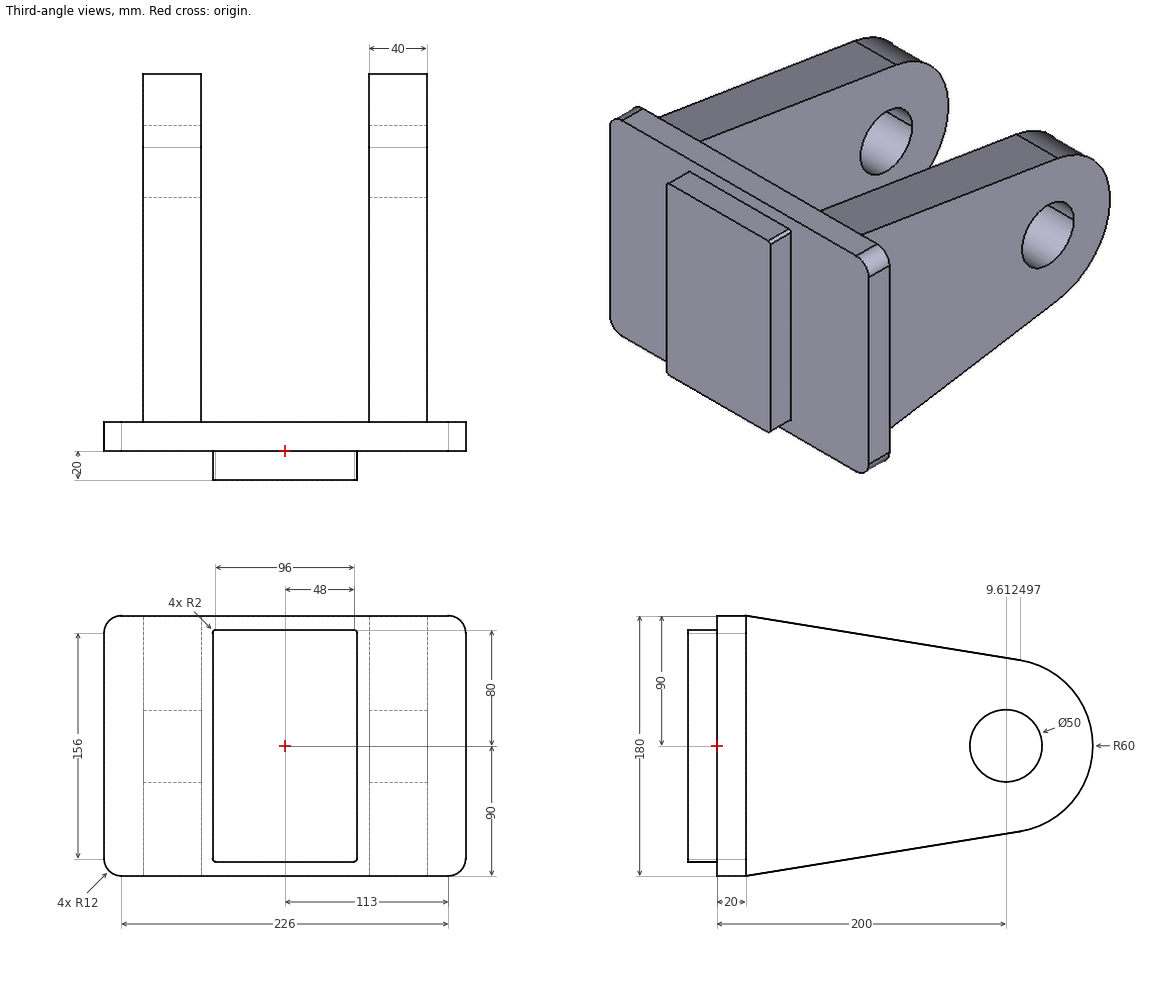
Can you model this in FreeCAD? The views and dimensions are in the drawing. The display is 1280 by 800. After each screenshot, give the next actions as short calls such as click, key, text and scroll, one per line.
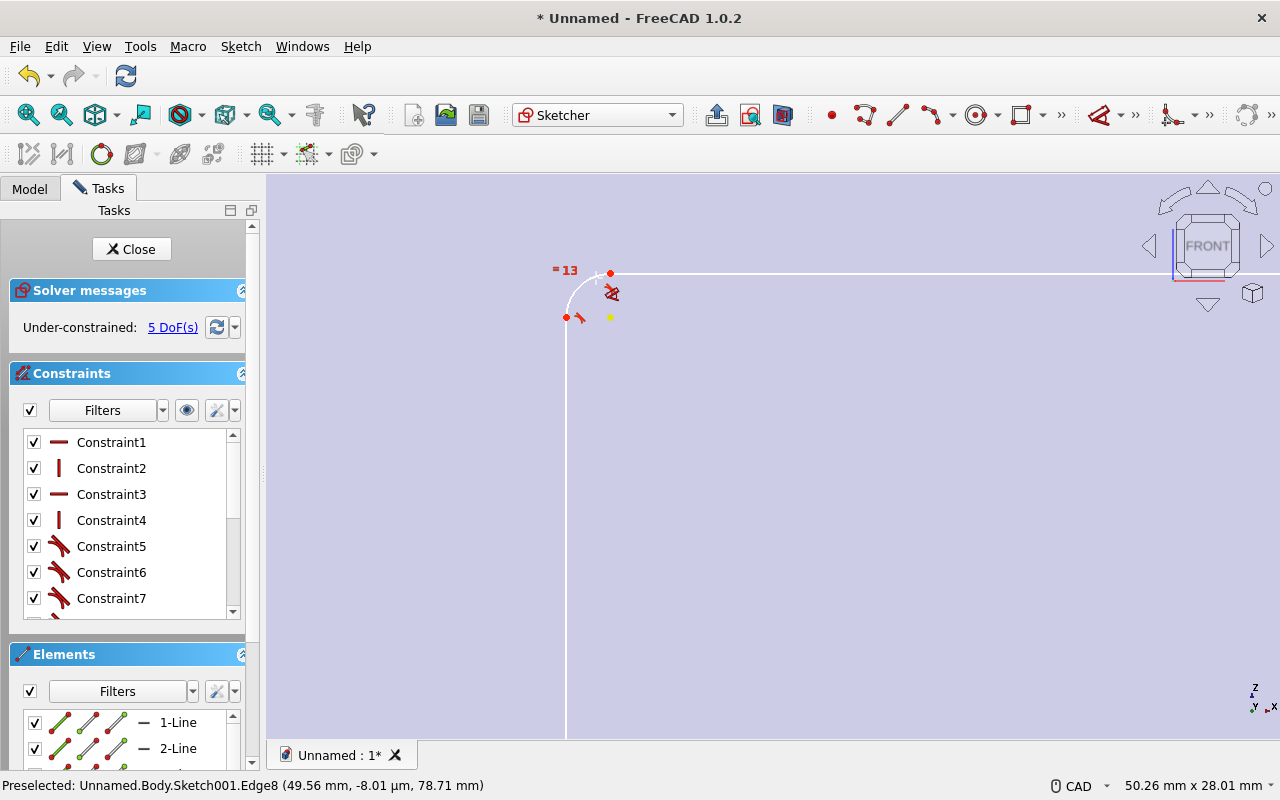
click(590, 279)
click(575, 251)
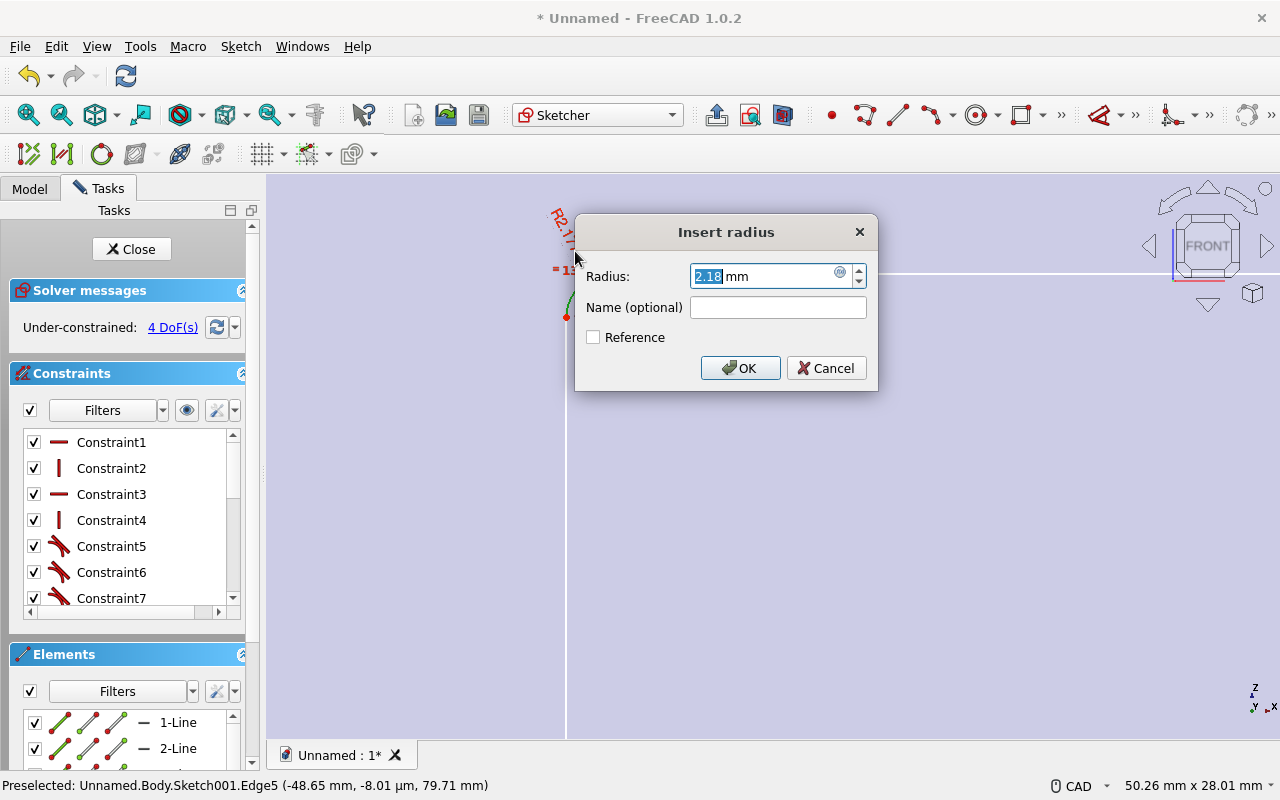
text(2)
key(Return)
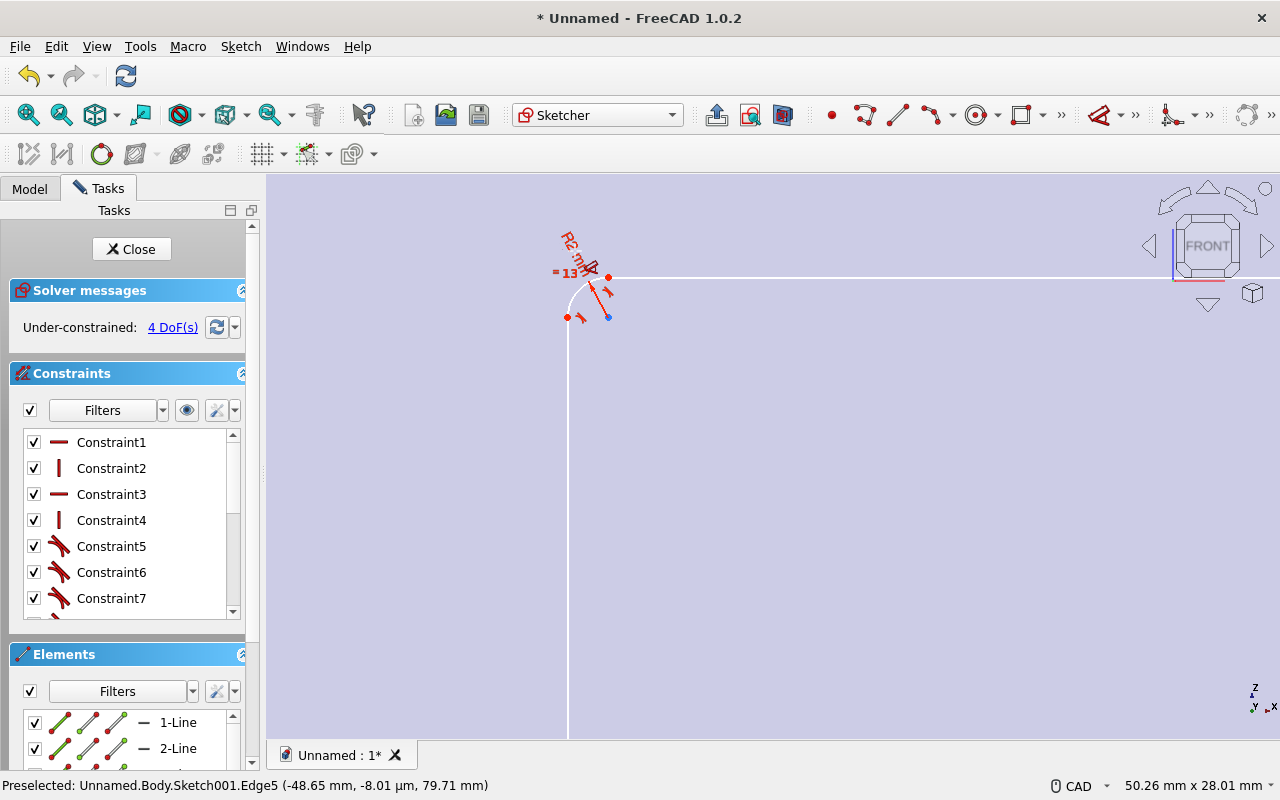
scroll(596, 278, down, 11)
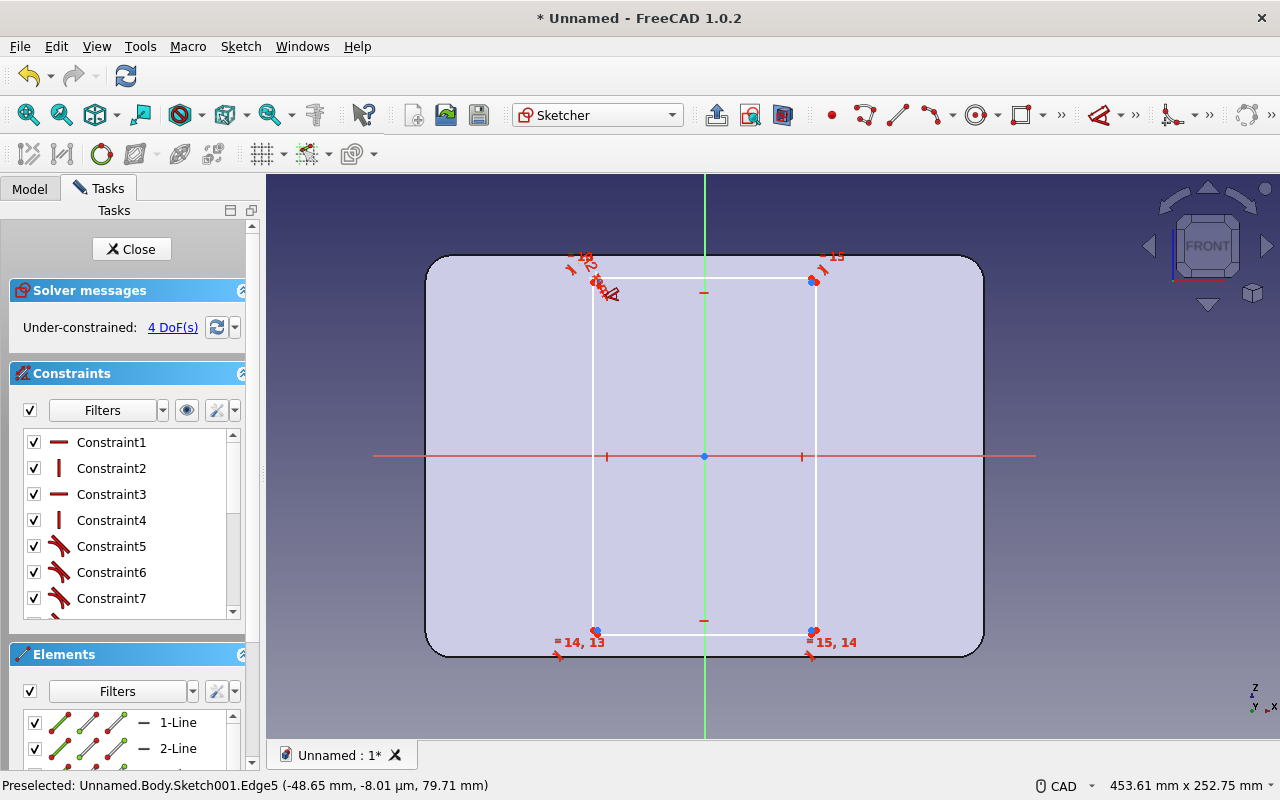
click(640, 278)
click(655, 244)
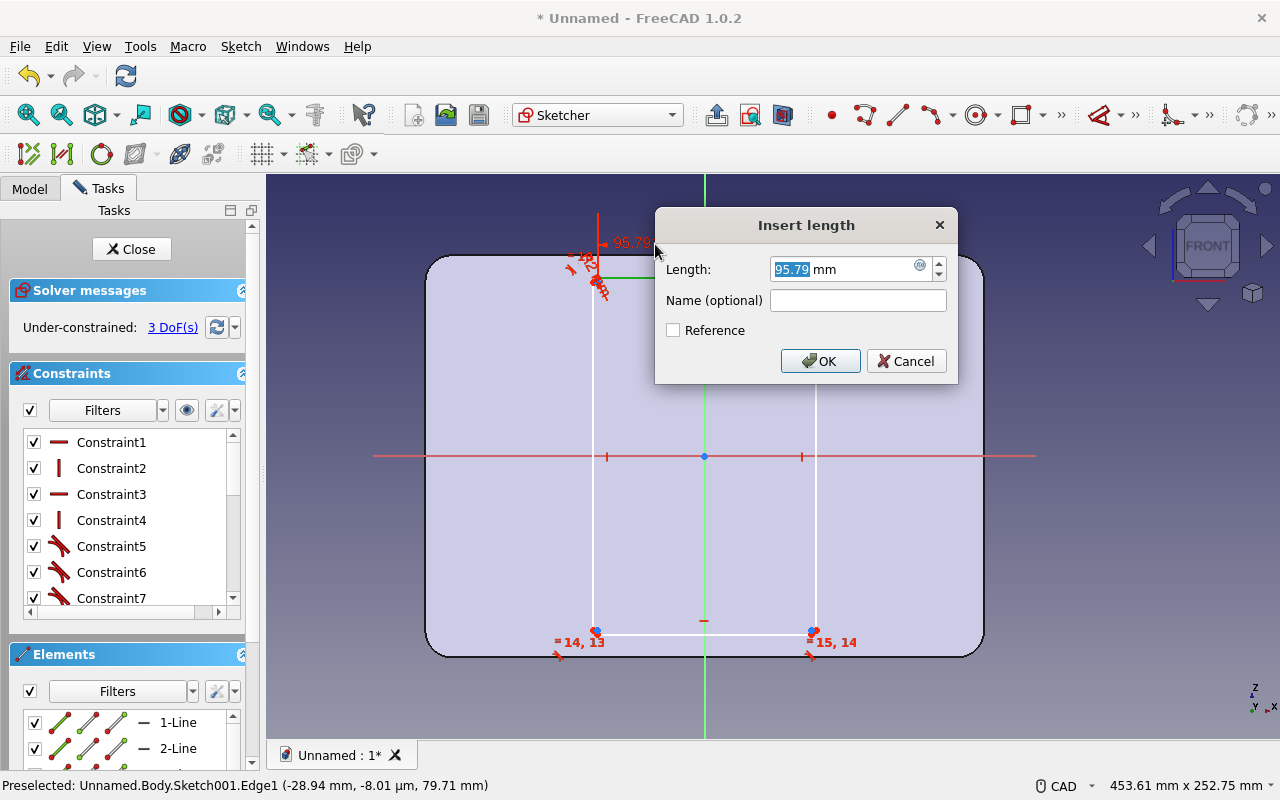
text(96)
key(Return)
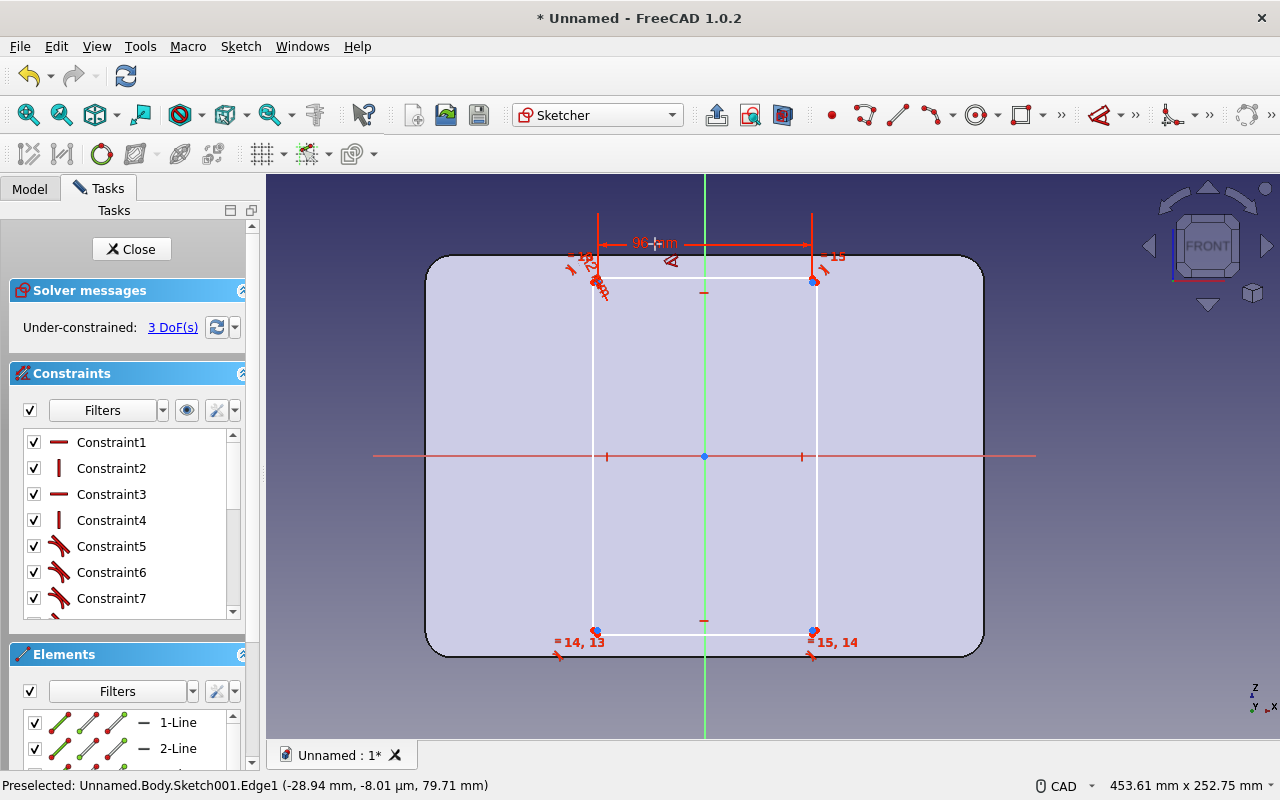
click(593, 387)
click(559, 377)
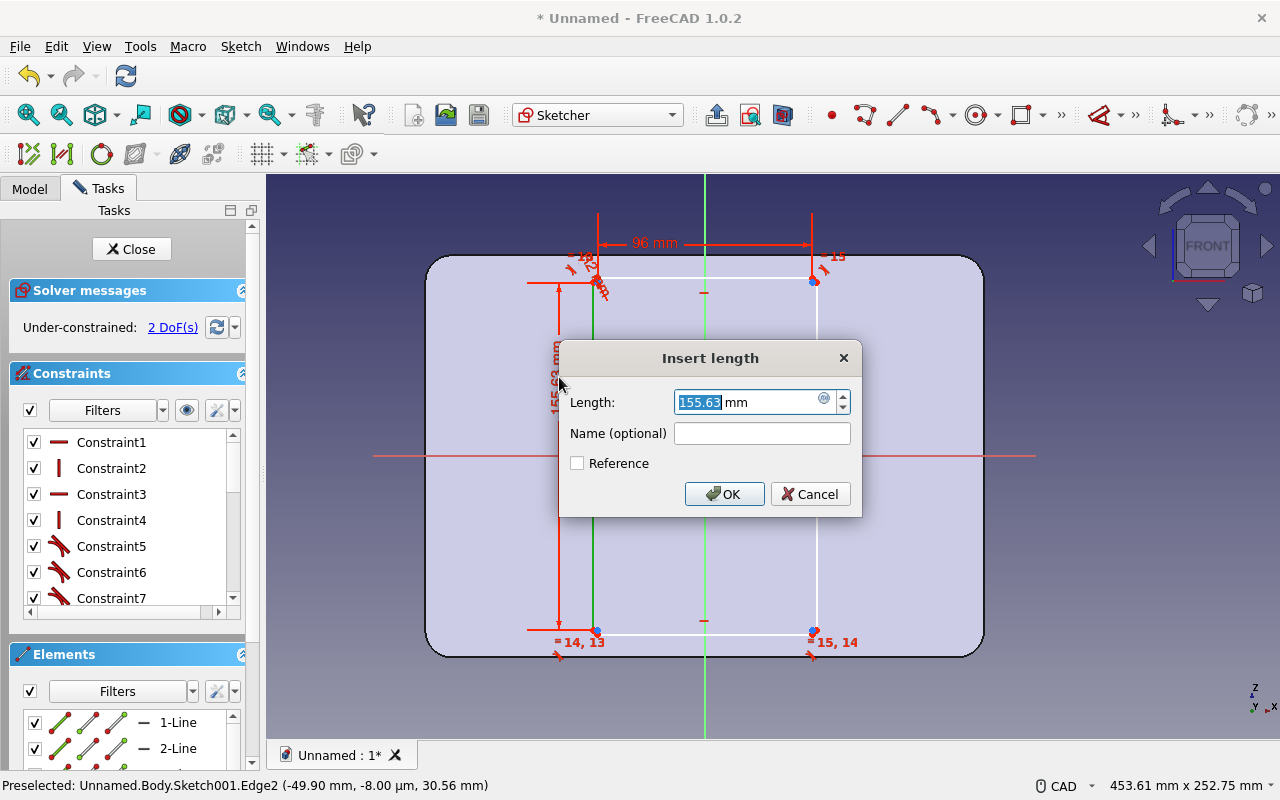
text(156)
key(Return)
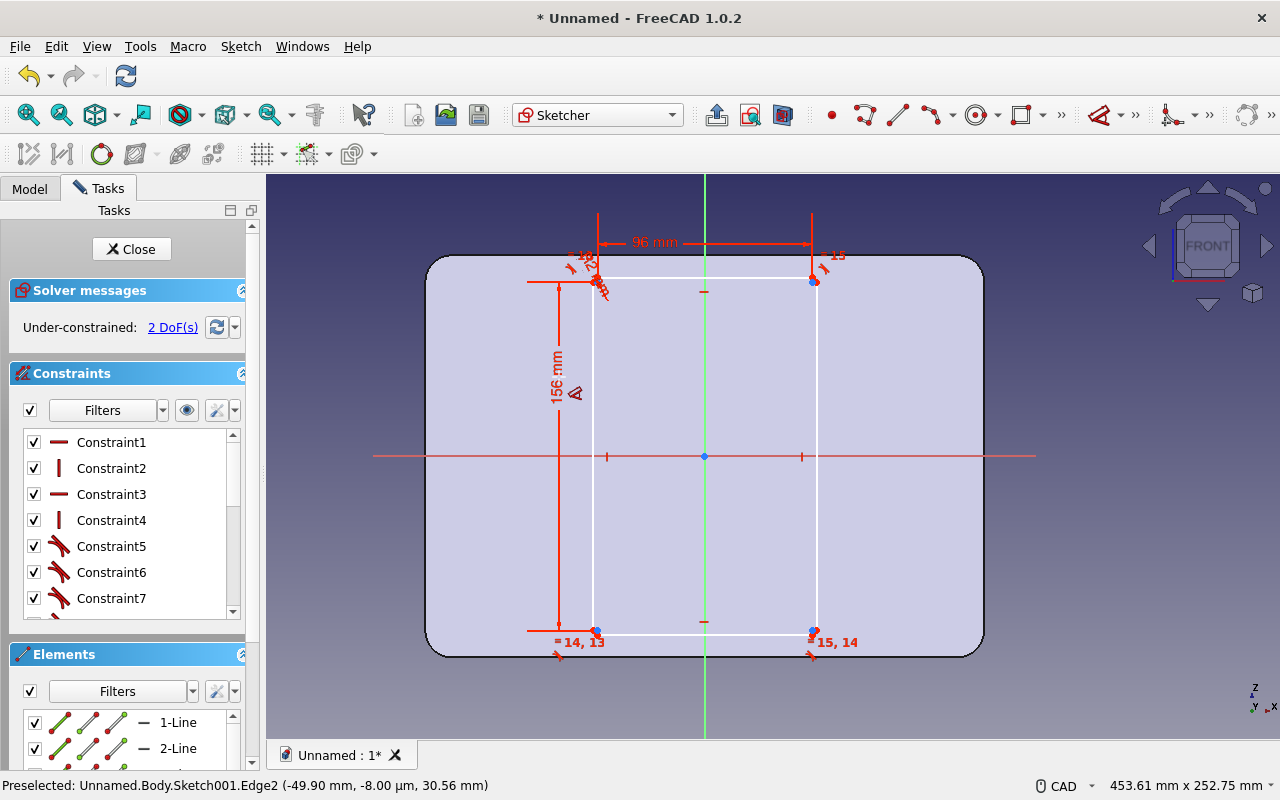
scroll(812, 278, up, 6)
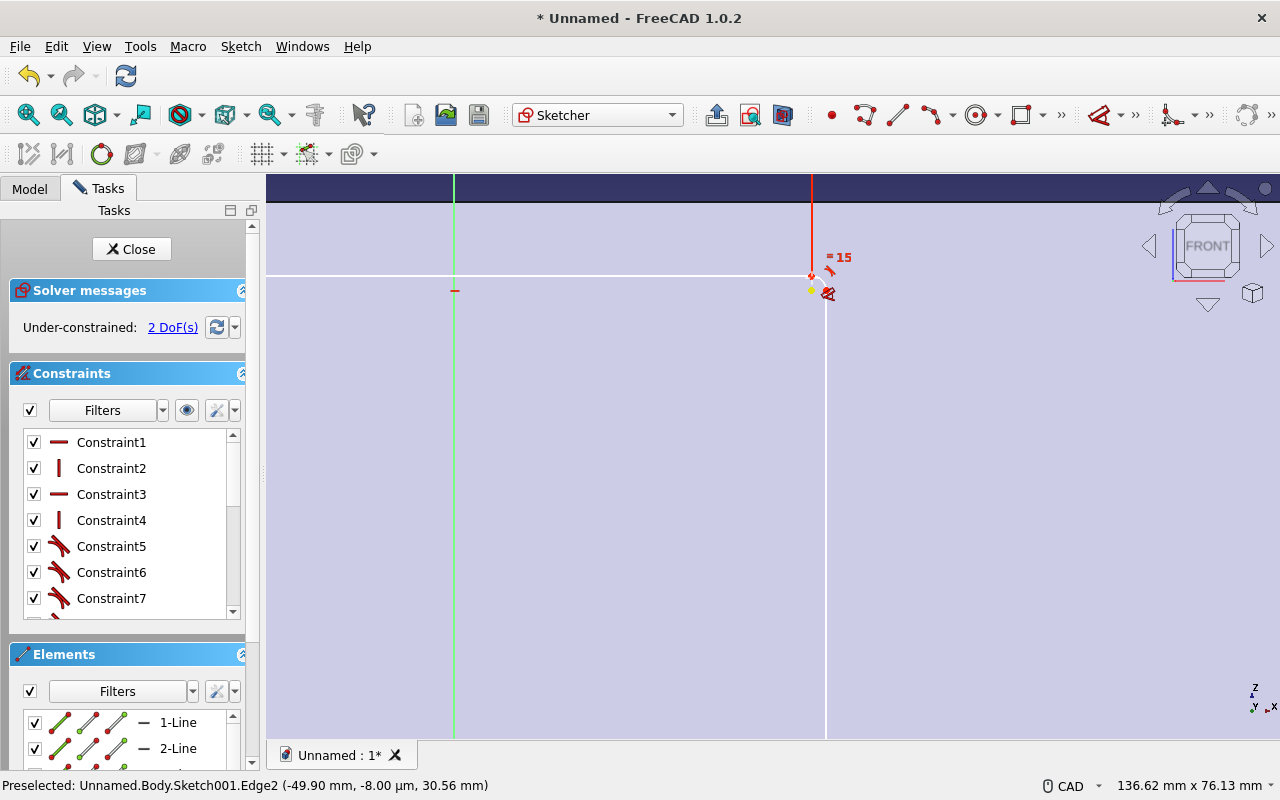
click(812, 276)
click(633, 242)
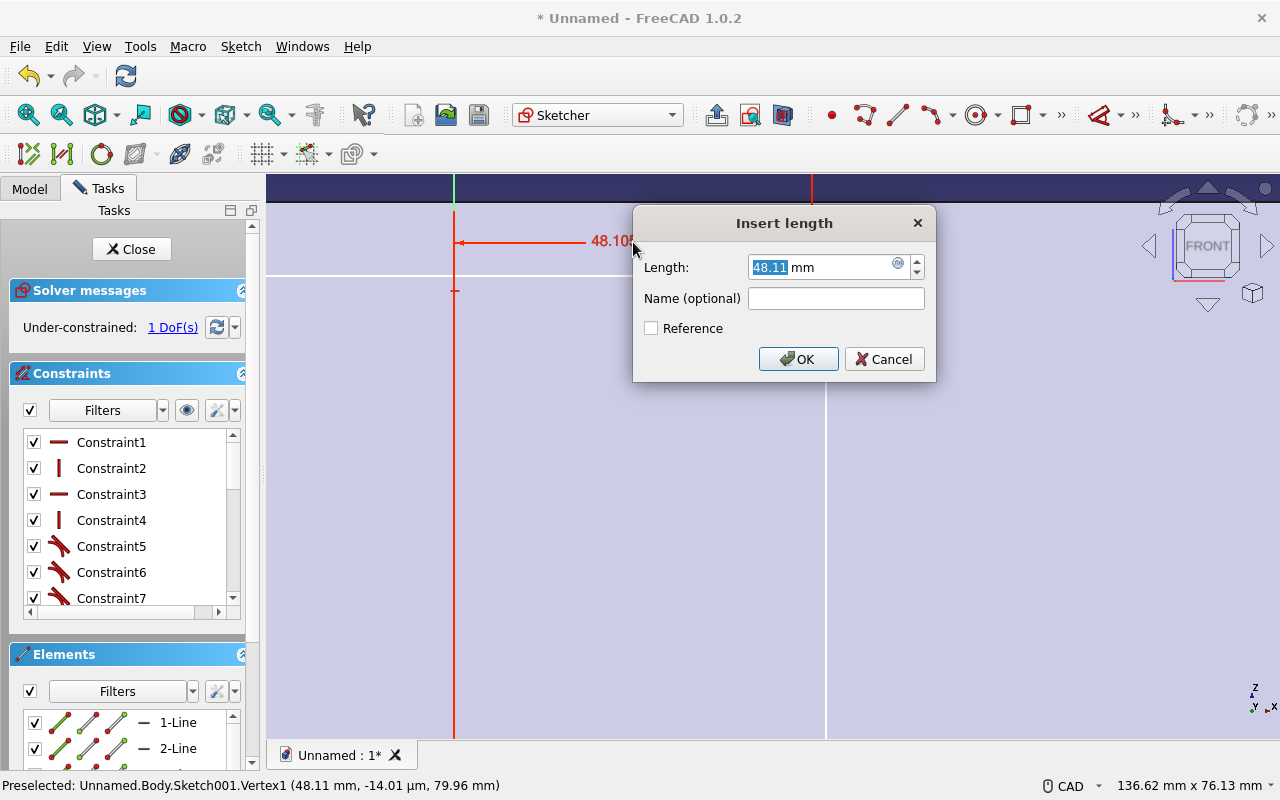
text(48)
key(Return)